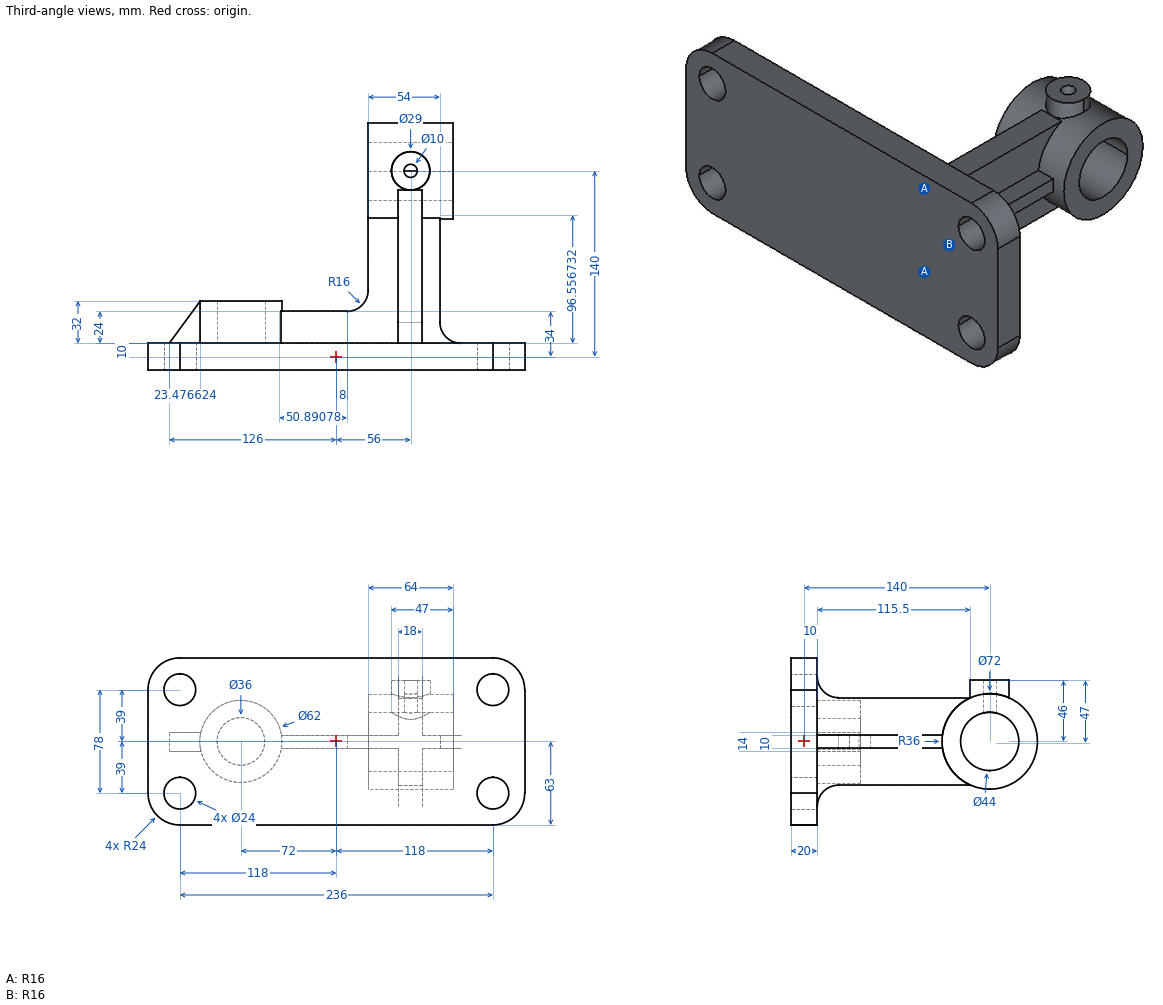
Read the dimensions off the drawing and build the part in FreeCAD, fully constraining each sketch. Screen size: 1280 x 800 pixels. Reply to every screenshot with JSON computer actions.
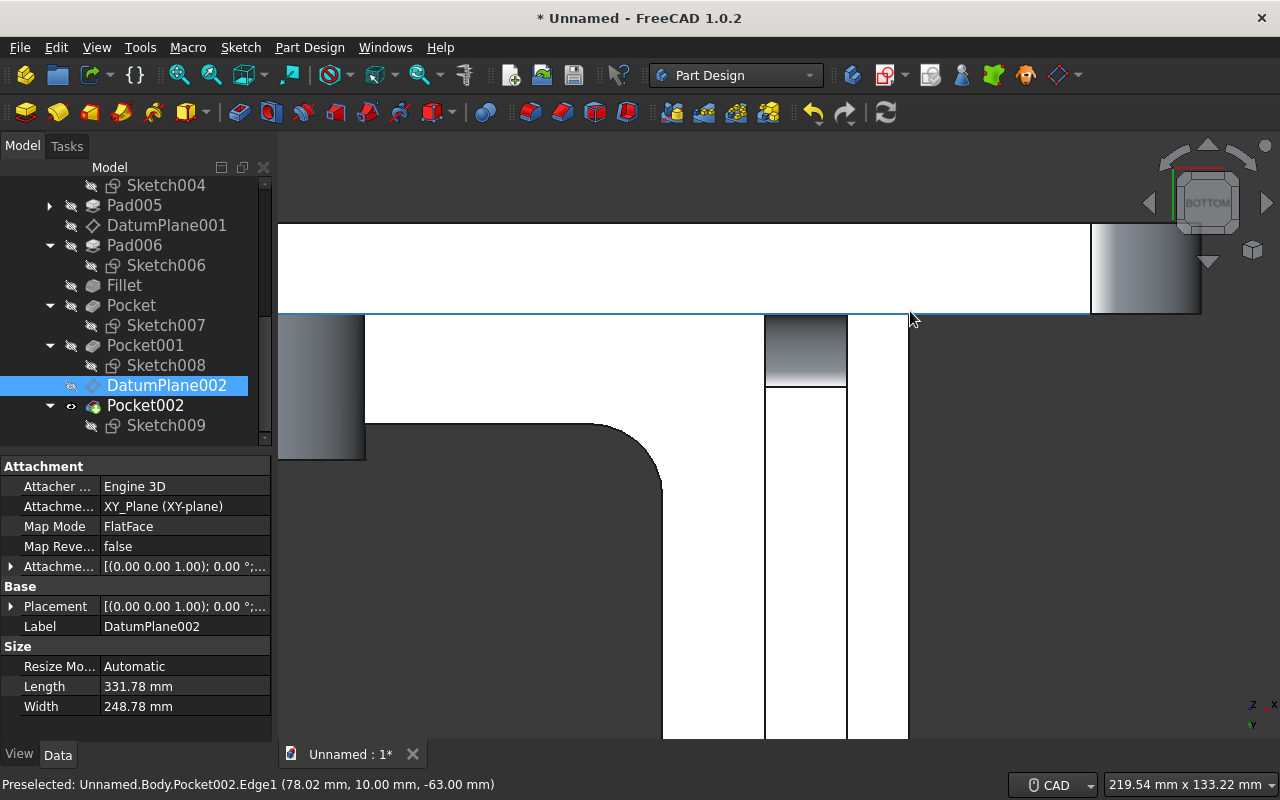
{"action": "left_click", "coordinate": [180, 76]}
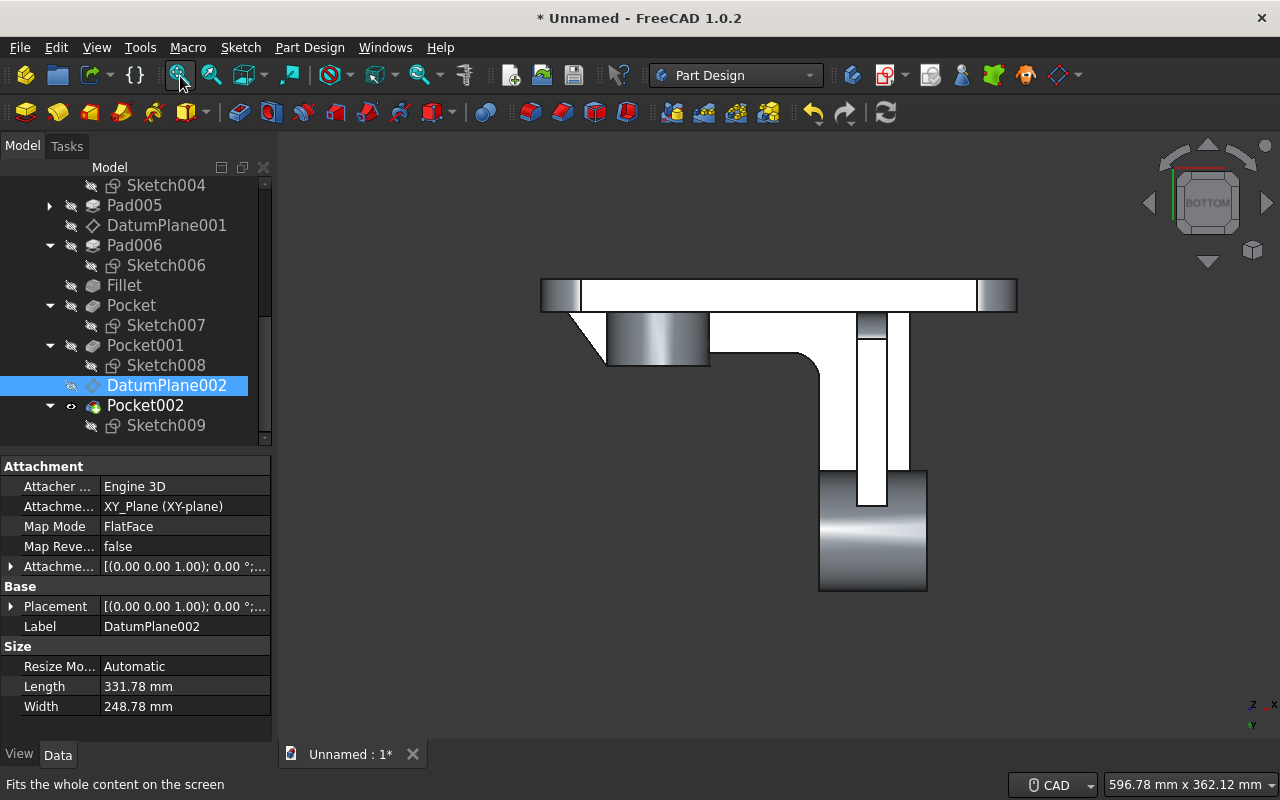
{"action": "key", "text": "4"}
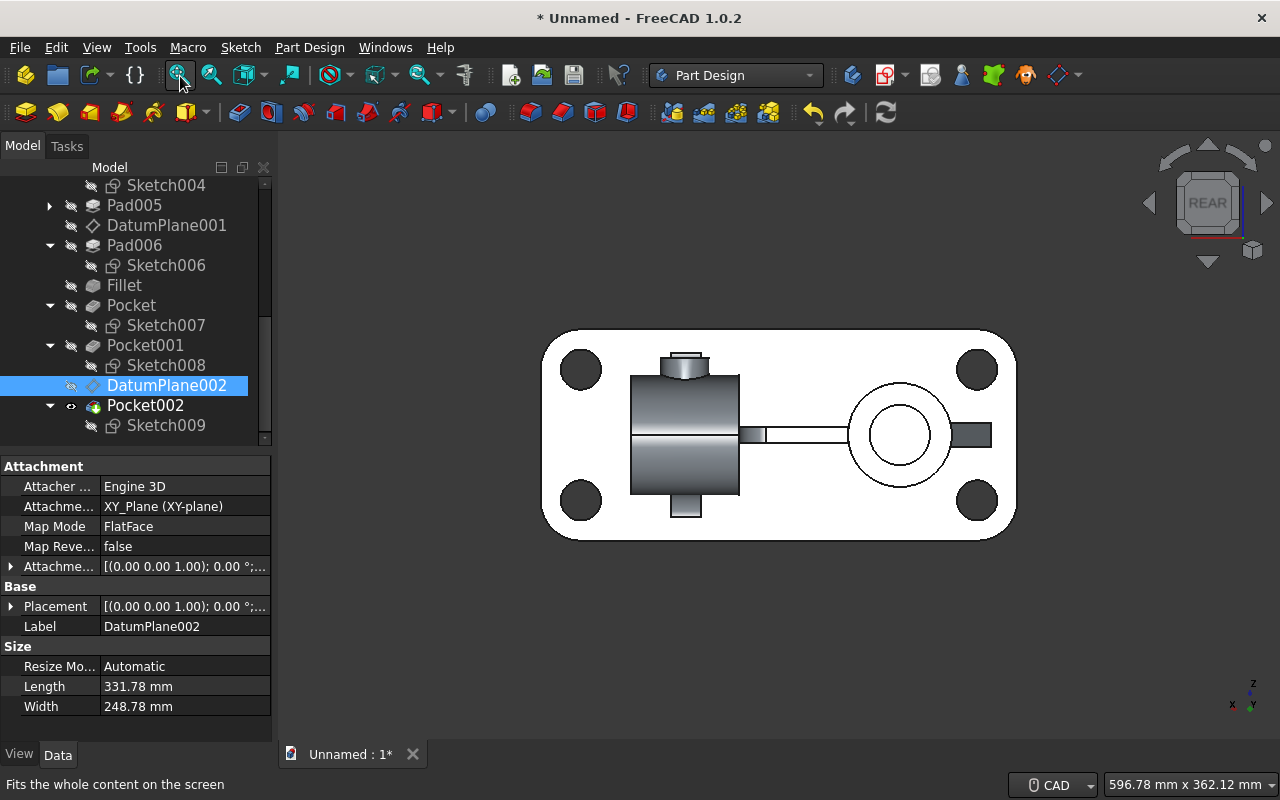
{"action": "scroll", "coordinate": [648, 434], "scroll_direction": "up", "scroll_amount": 5}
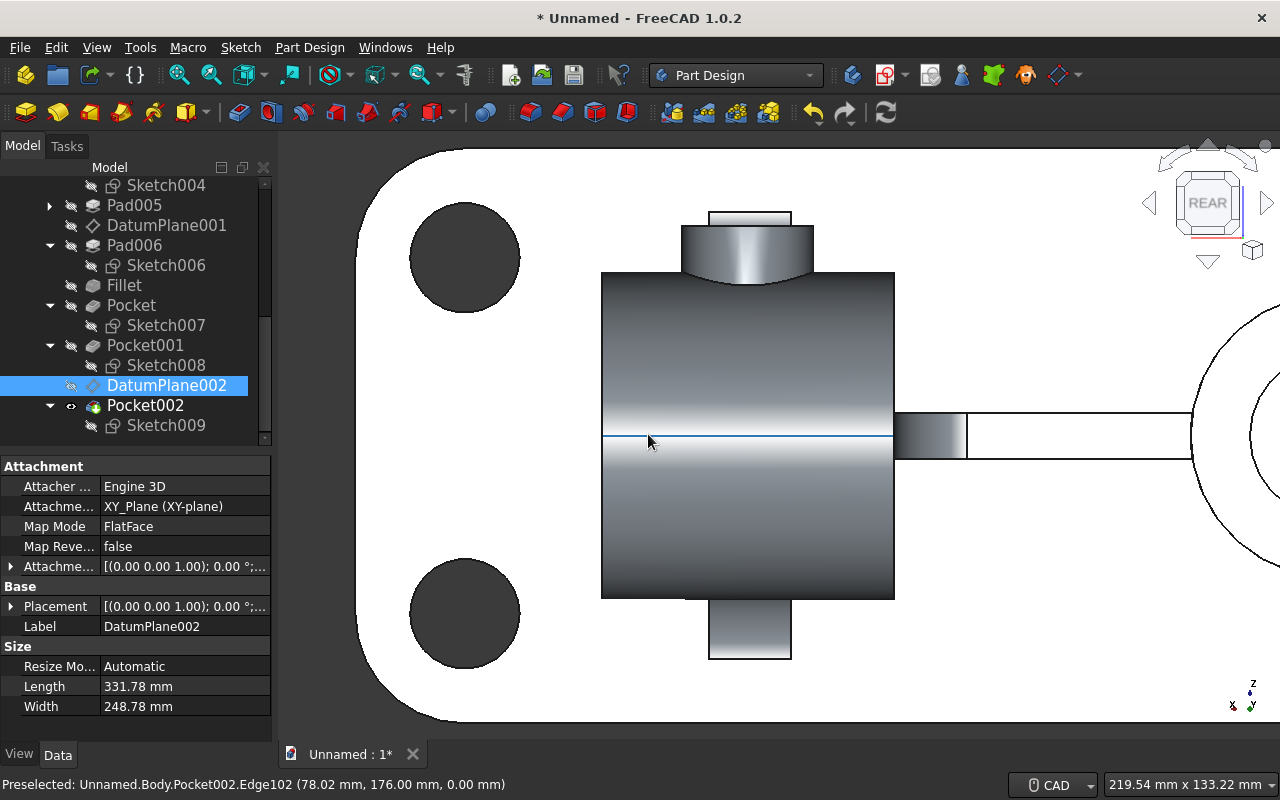
{"action": "left_click", "coordinate": [180, 76]}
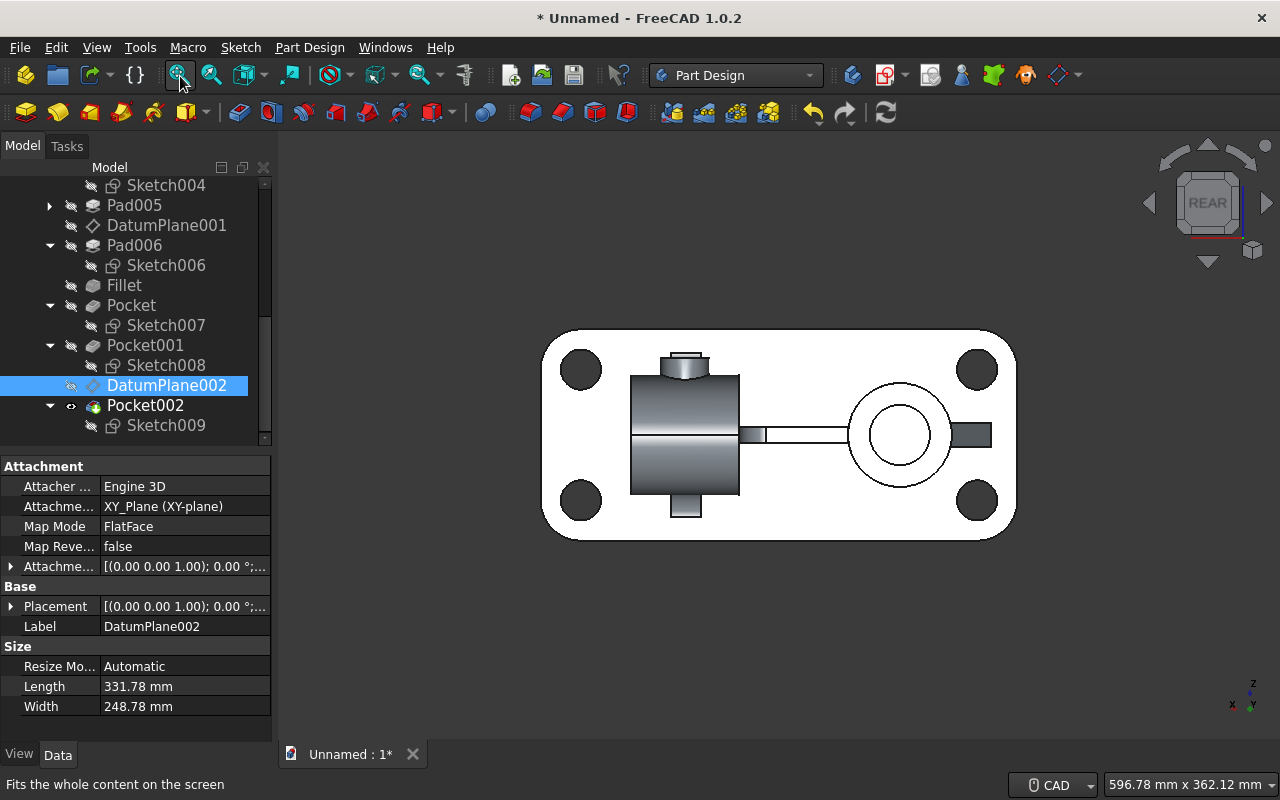
{"action": "key", "text": "6"}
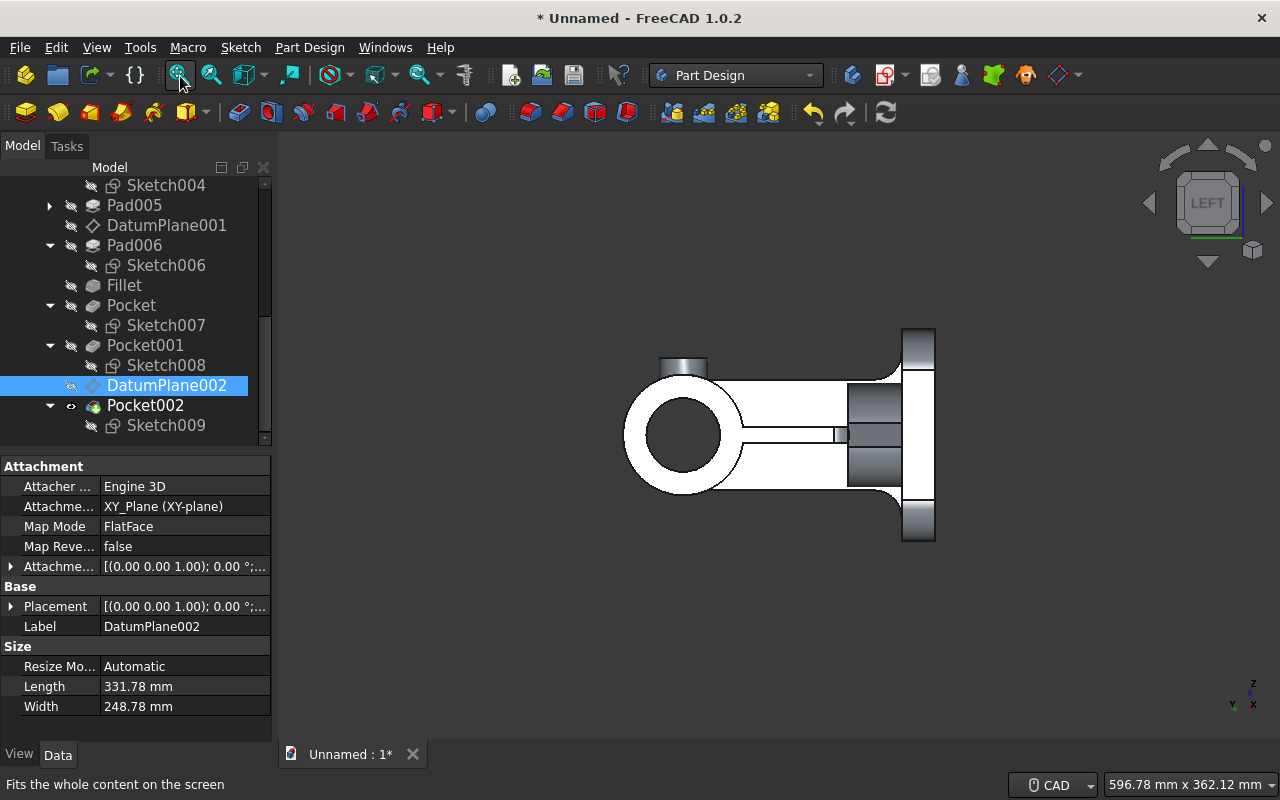
{"action": "left_click", "coordinate": [180, 76]}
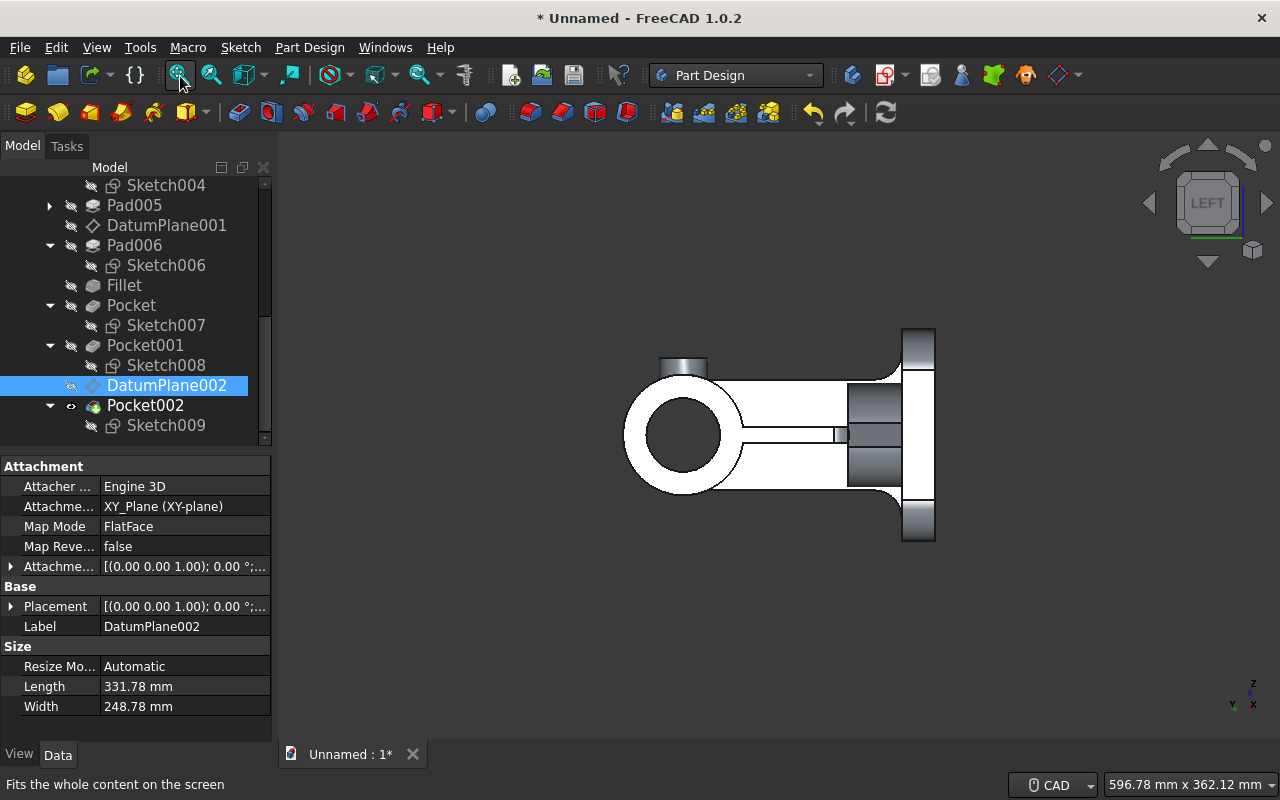
{"action": "scroll", "coordinate": [902, 434], "scroll_direction": "up", "scroll_amount": 5}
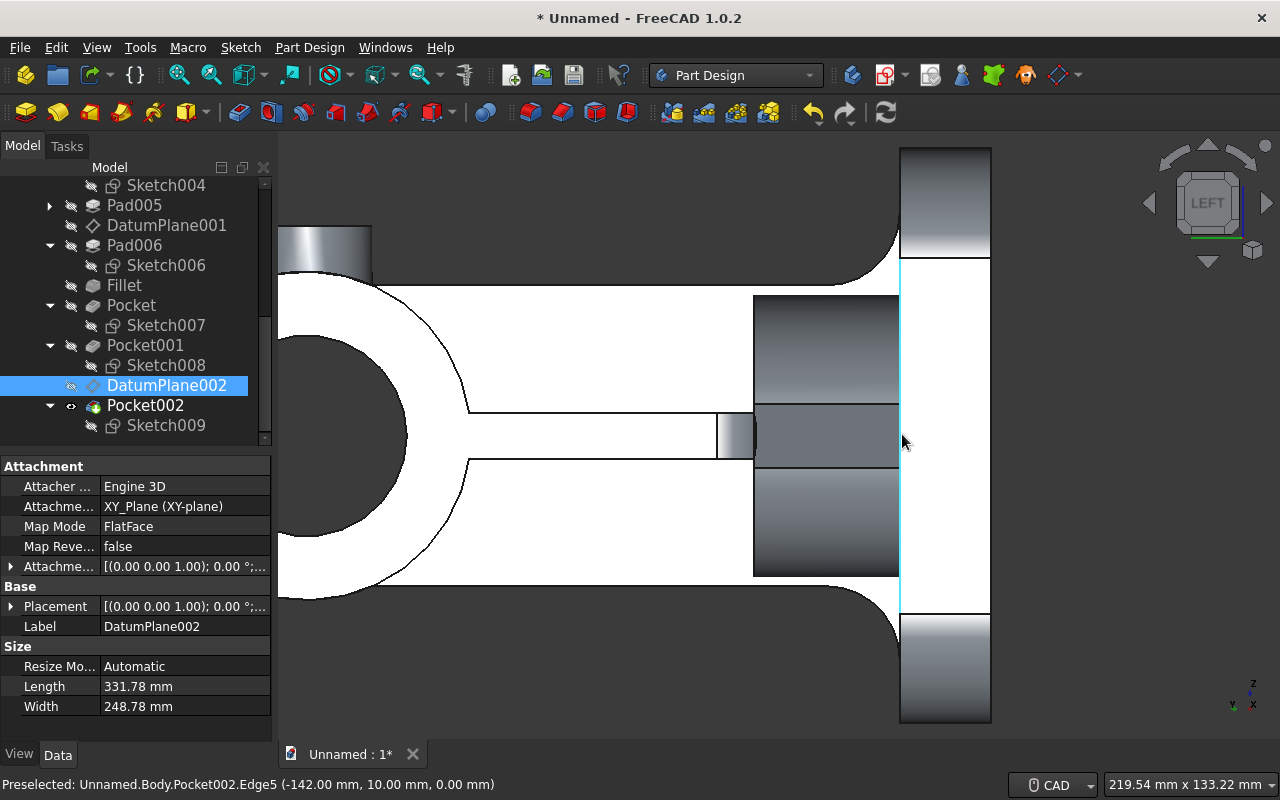
{"action": "left_click", "coordinate": [180, 76]}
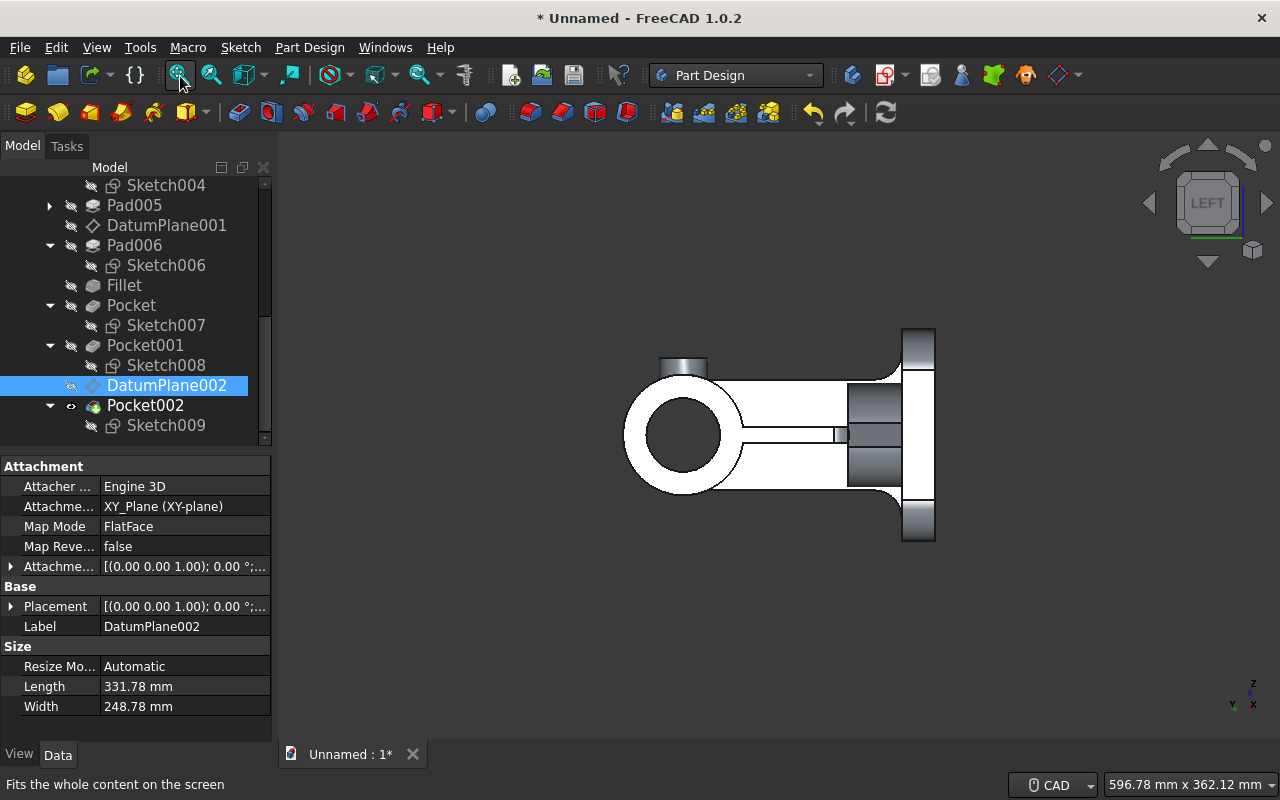
{"action": "key", "text": "v 3"}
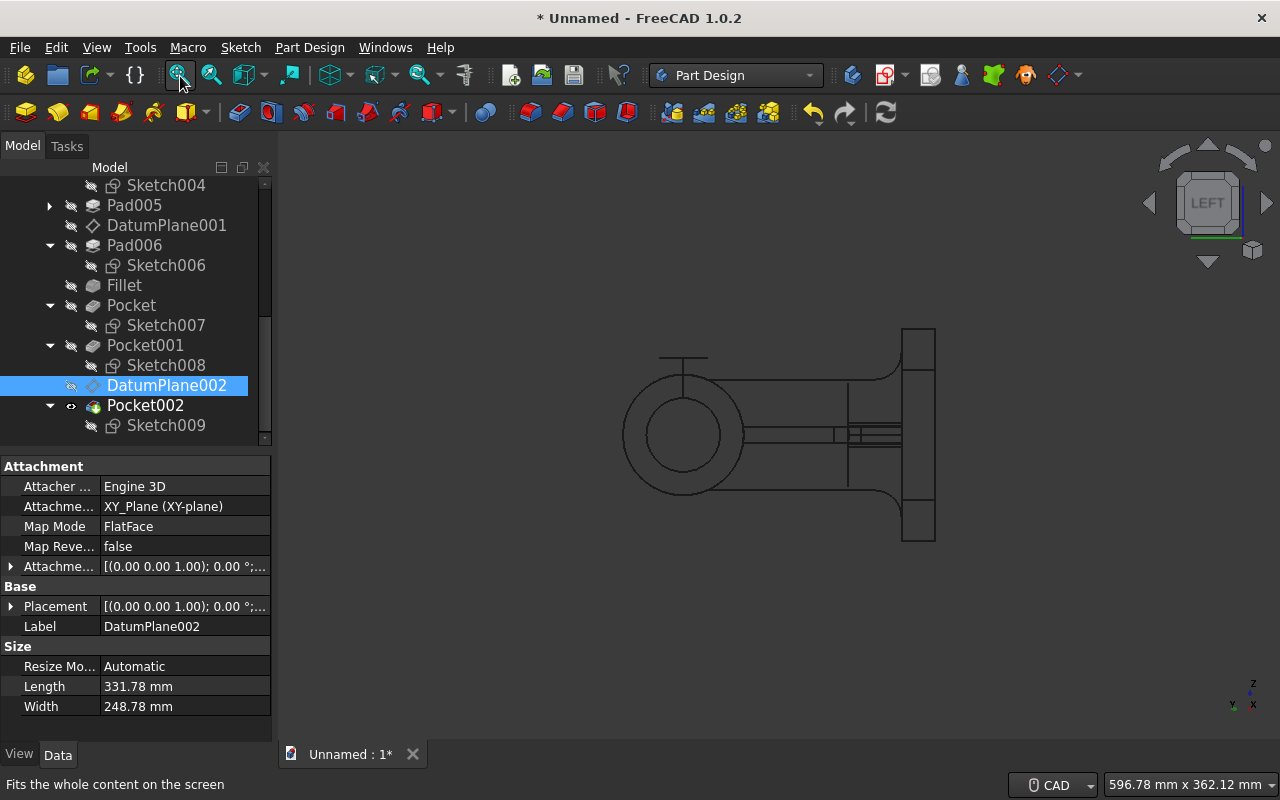
{"action": "key", "text": "0"}